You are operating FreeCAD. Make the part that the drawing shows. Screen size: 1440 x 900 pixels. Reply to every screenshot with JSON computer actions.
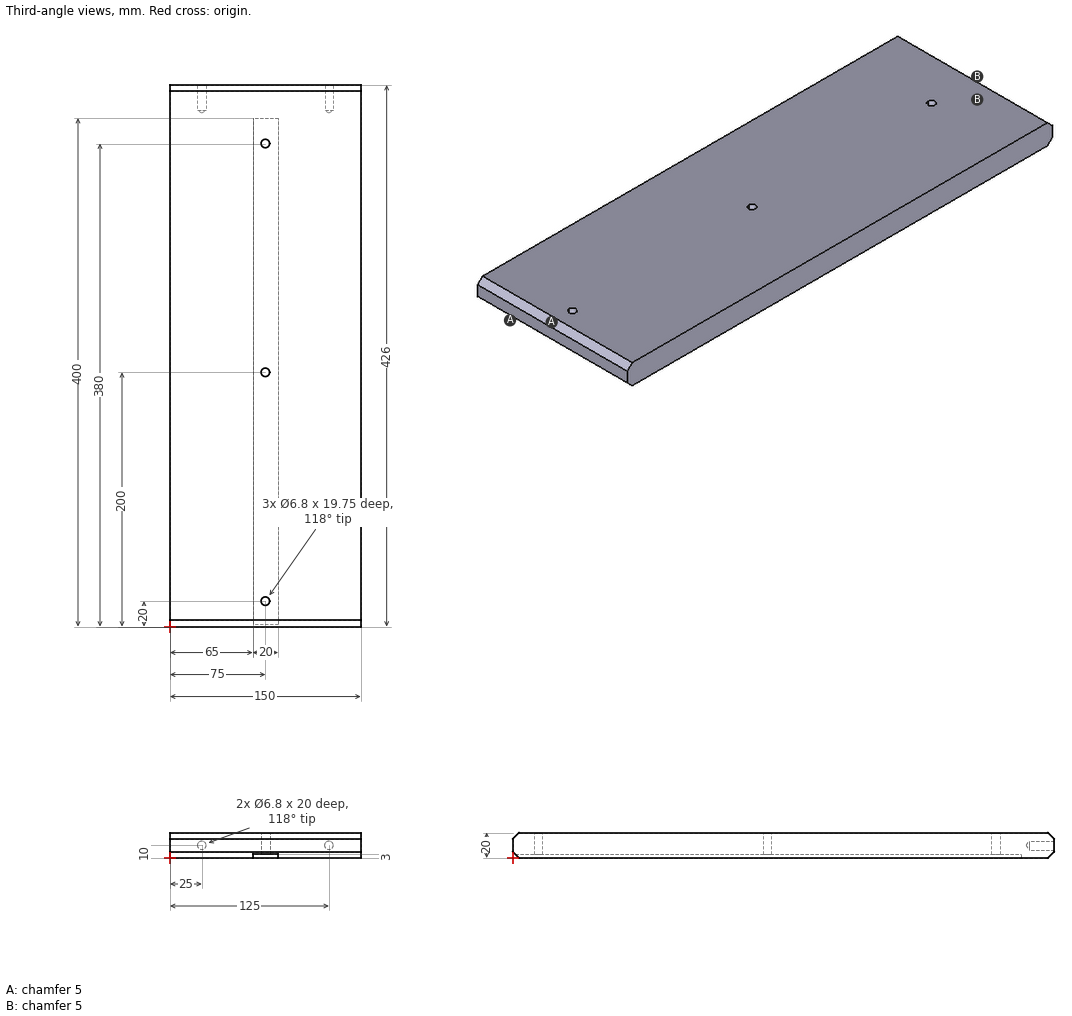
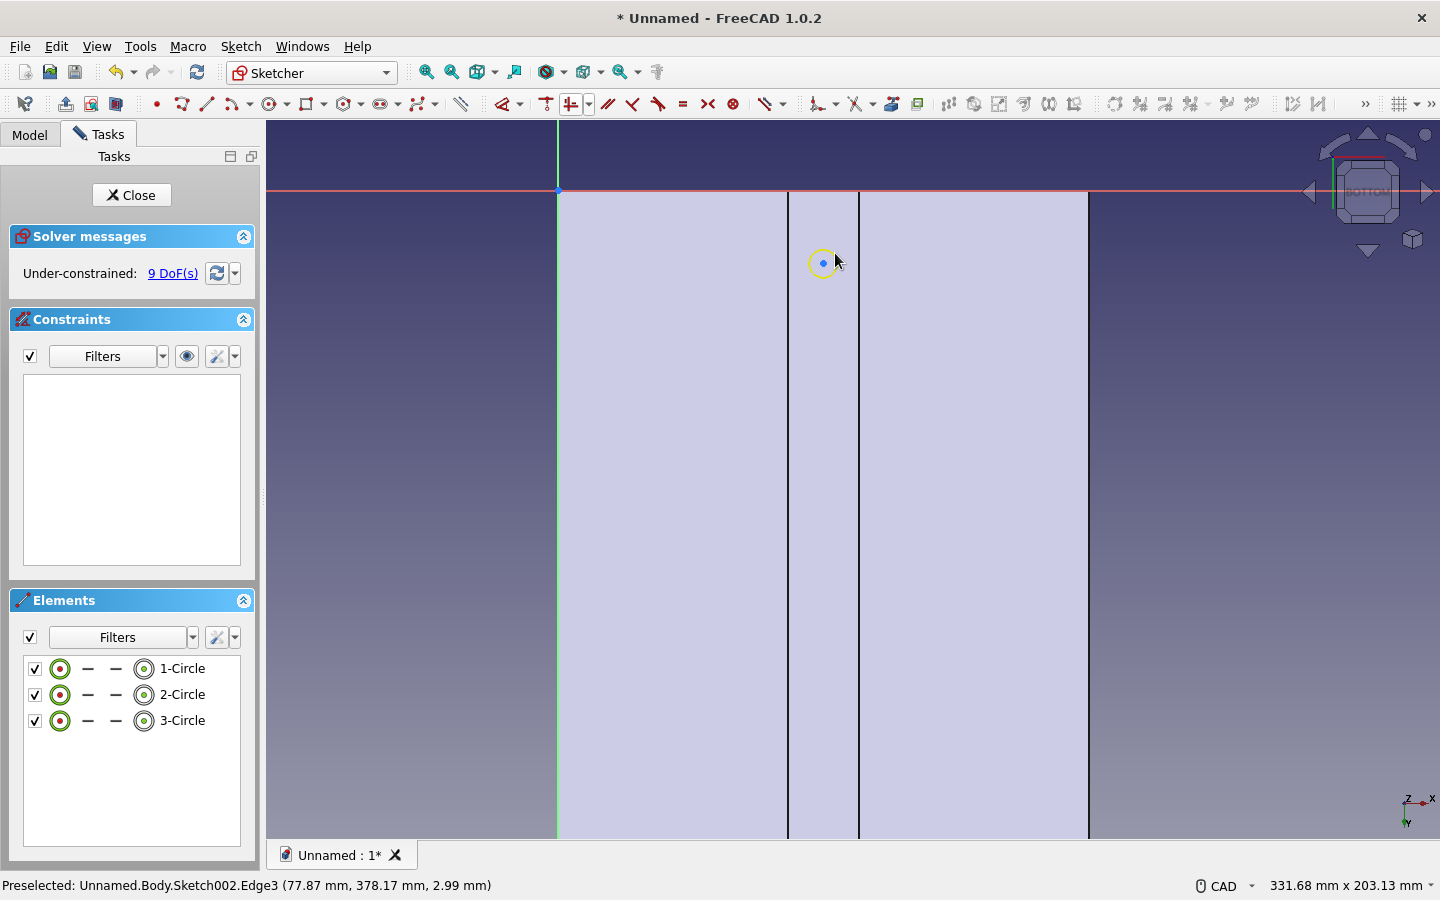
{"action": "left_click", "coordinate": [833, 254]}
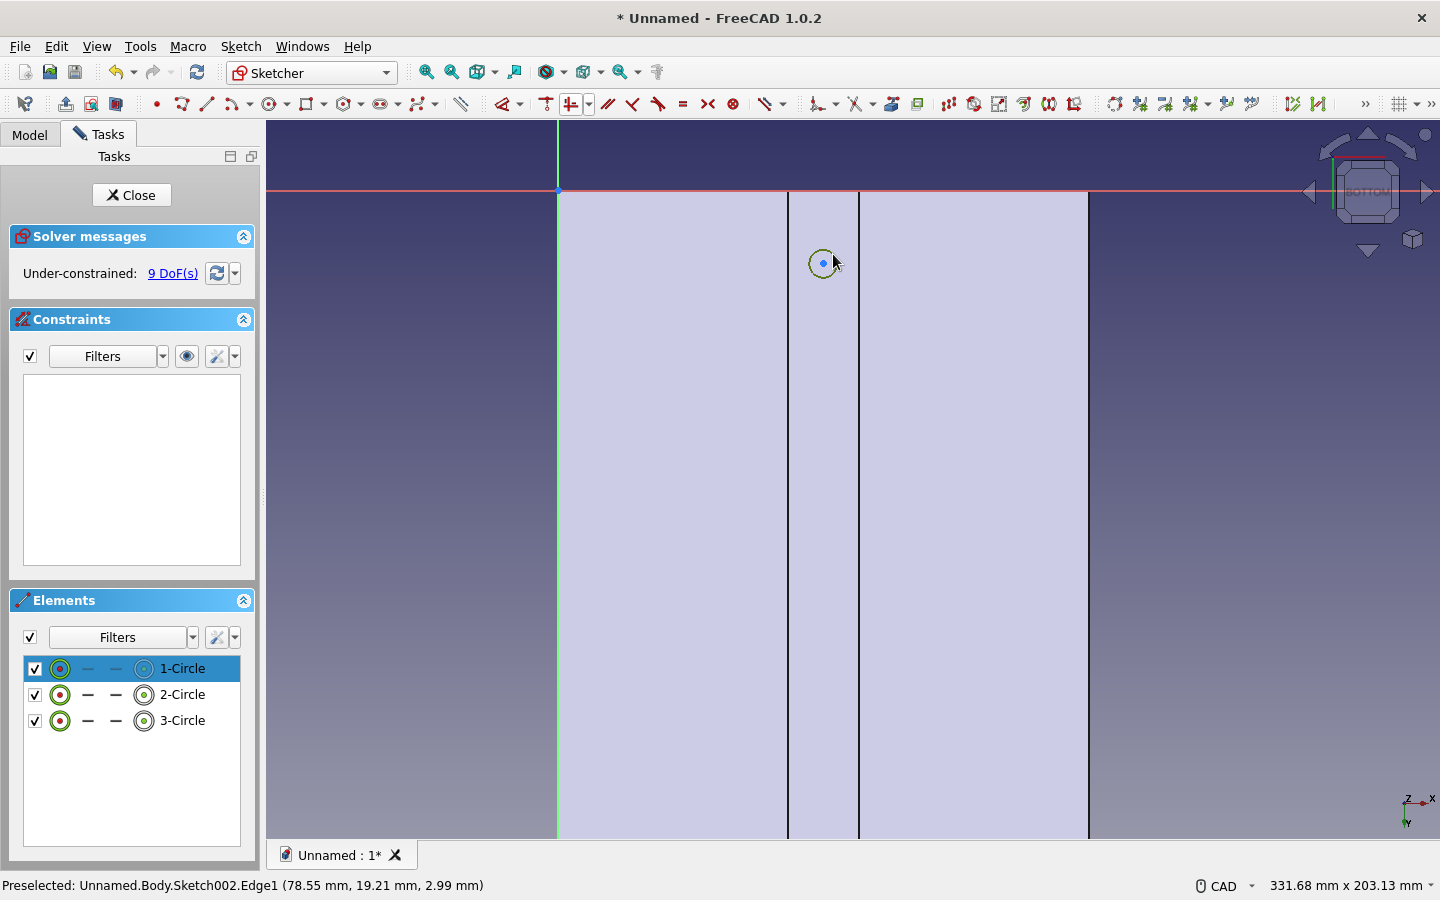
{"action": "scroll", "coordinate": [835, 253], "scroll_direction": "down", "scroll_amount": 5}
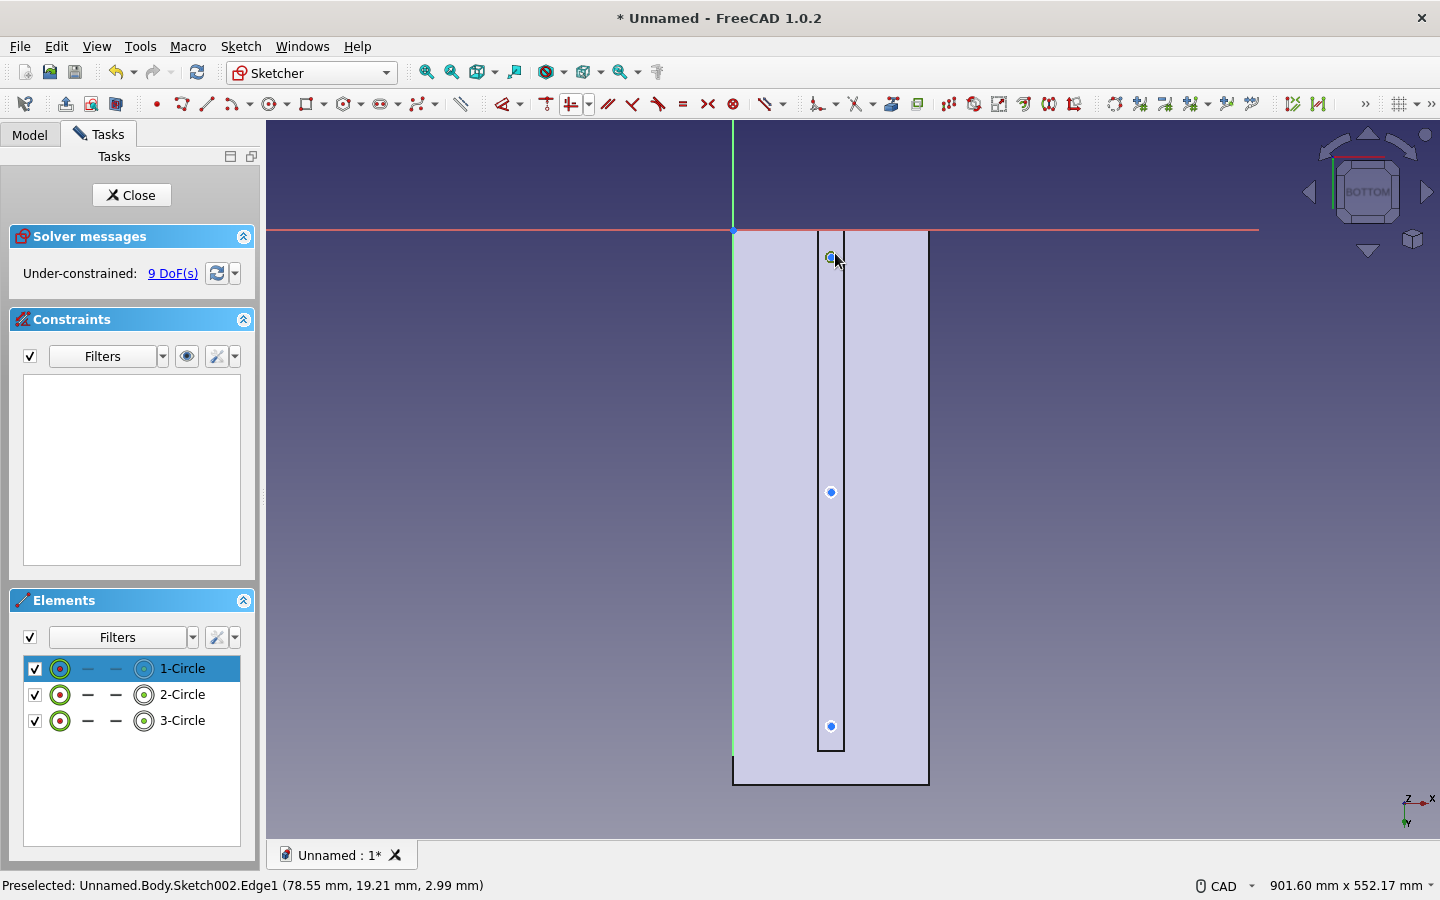
{"action": "scroll", "coordinate": [835, 488], "scroll_direction": "up", "scroll_amount": 5}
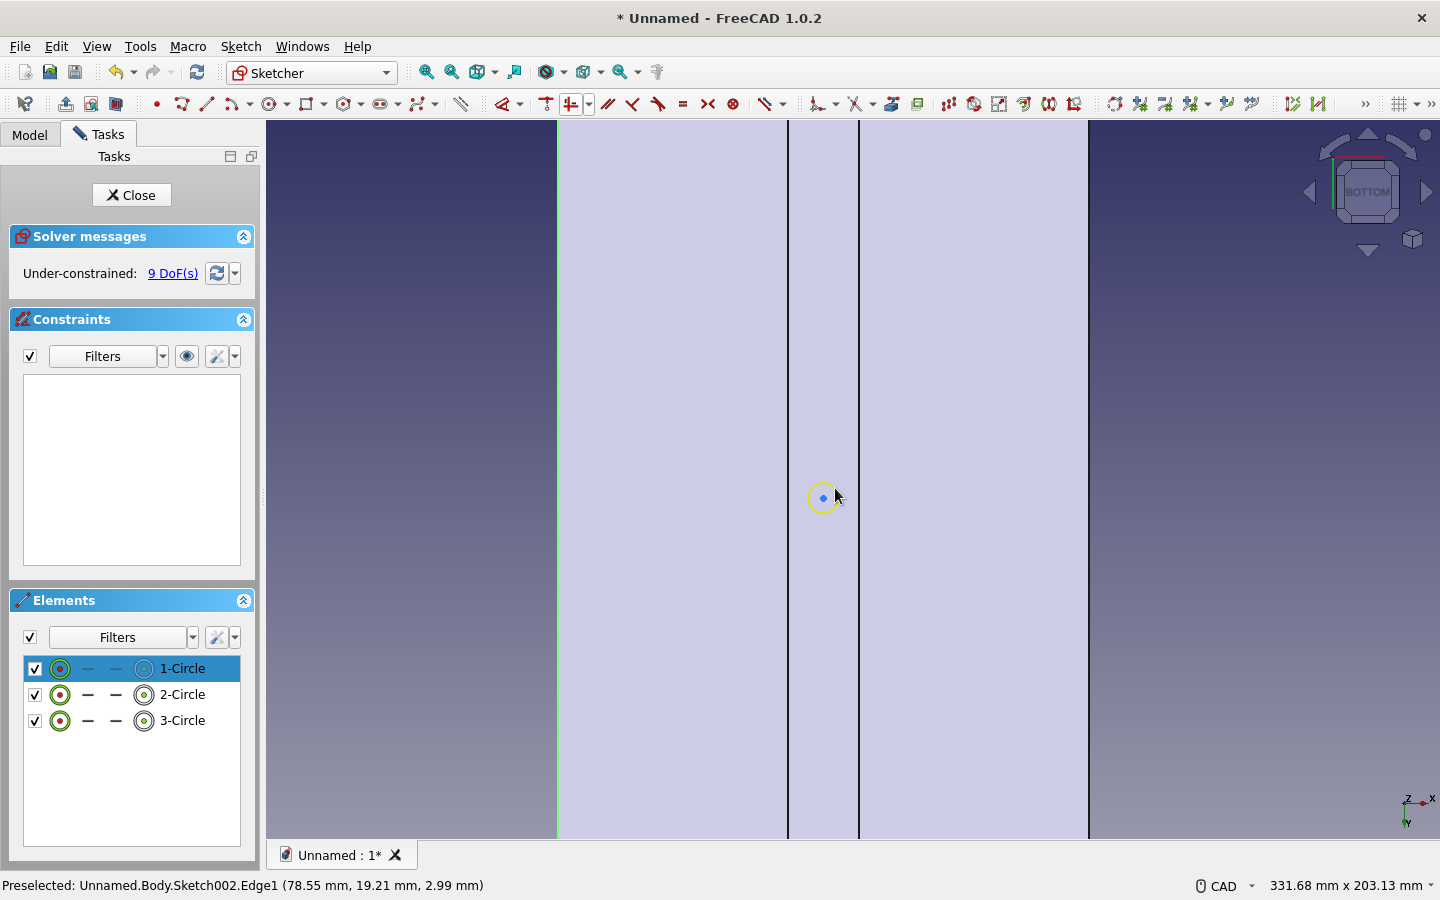
{"action": "left_click", "coordinate": [834, 488]}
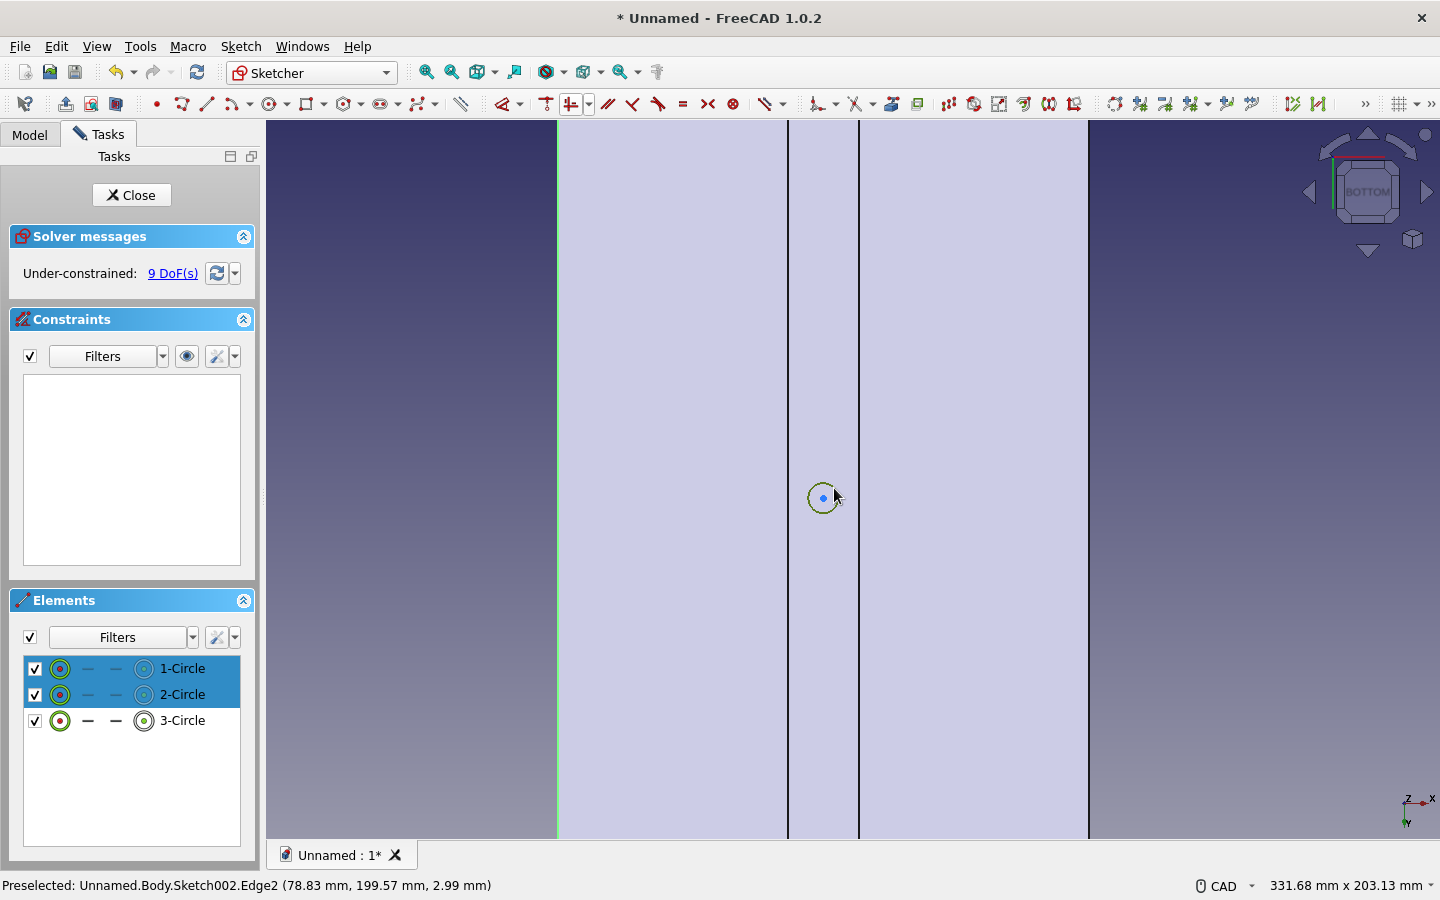
{"action": "scroll", "coordinate": [835, 488], "scroll_direction": "down", "scroll_amount": 5}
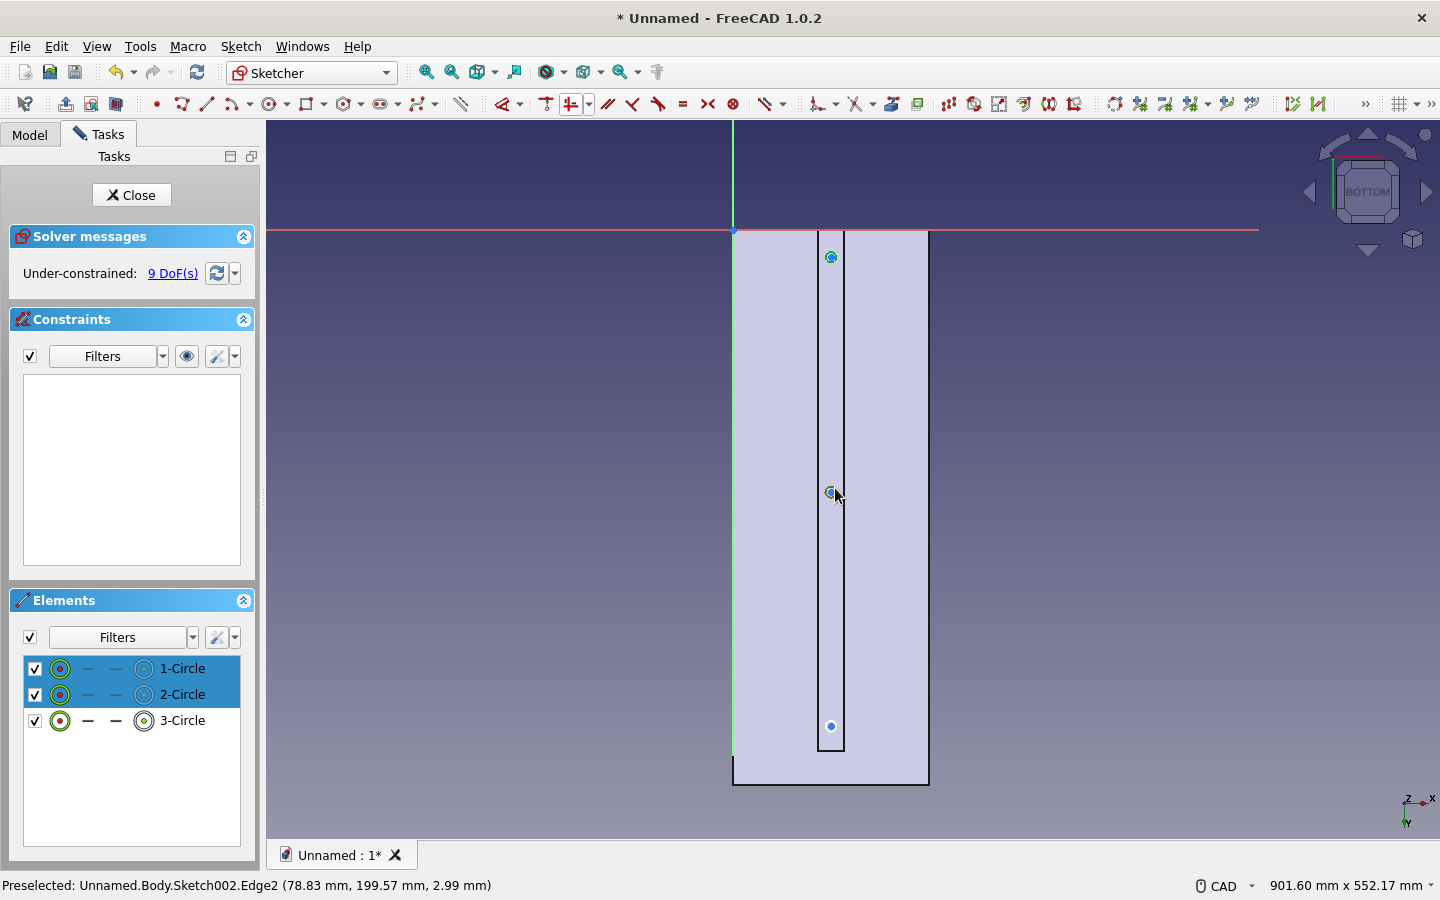
{"action": "scroll", "coordinate": [835, 722], "scroll_direction": "up", "scroll_amount": 5}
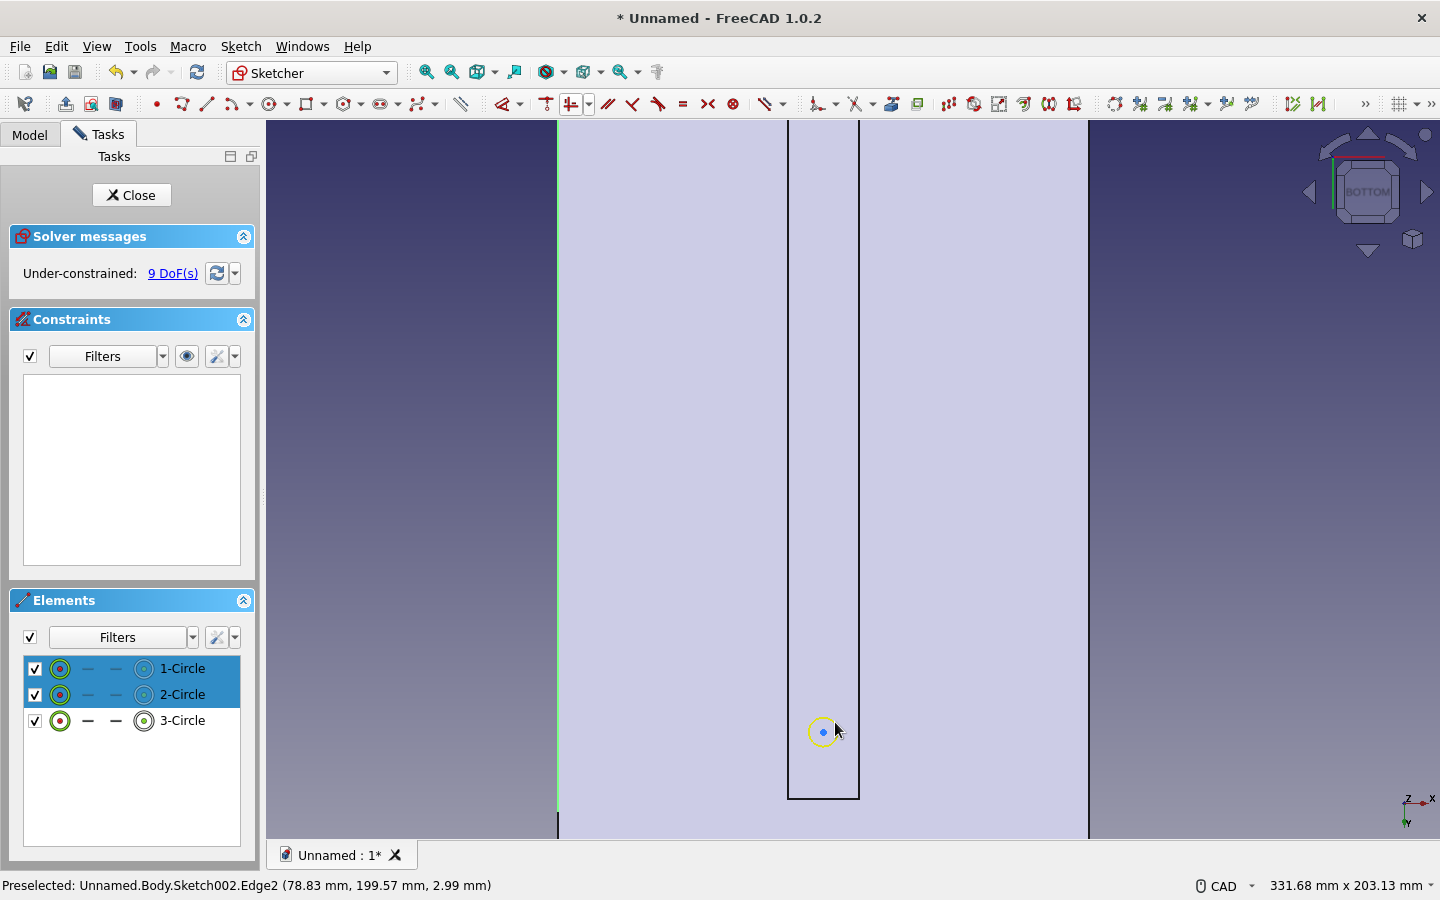
{"action": "left_click", "coordinate": [833, 722]}